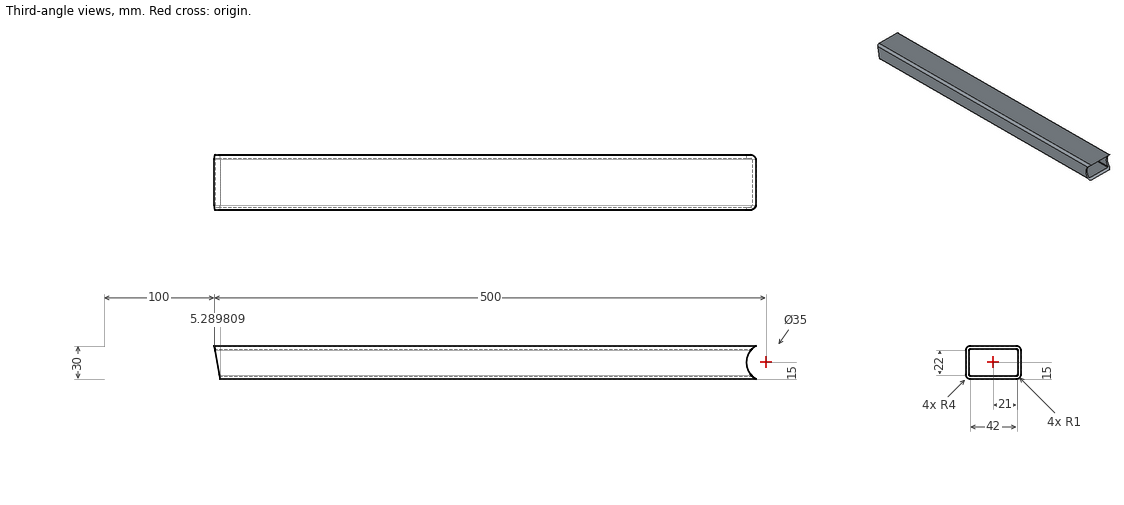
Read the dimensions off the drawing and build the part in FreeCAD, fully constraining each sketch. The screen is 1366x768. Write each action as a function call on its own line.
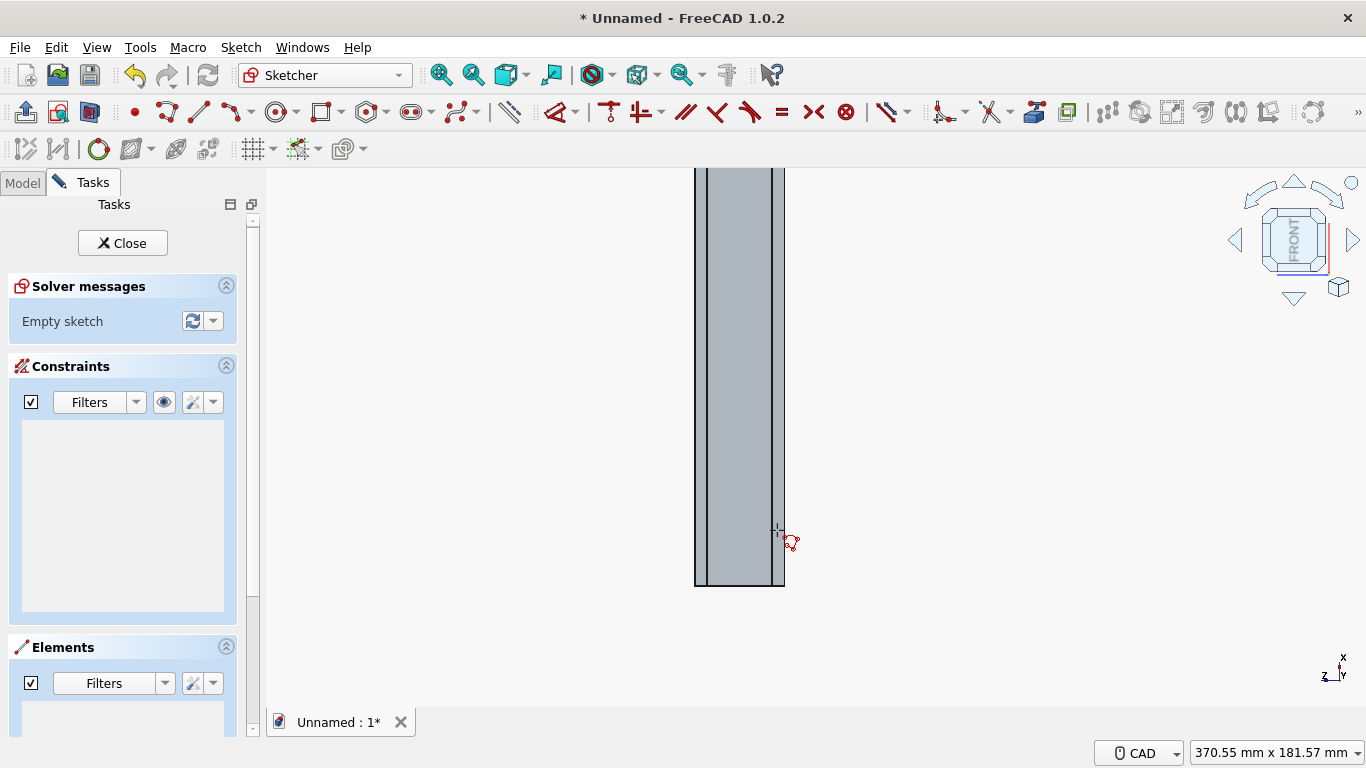
click(784, 274)
click(695, 289)
click(695, 586)
click(784, 586)
click(784, 275)
key(Escape)
key(Escape)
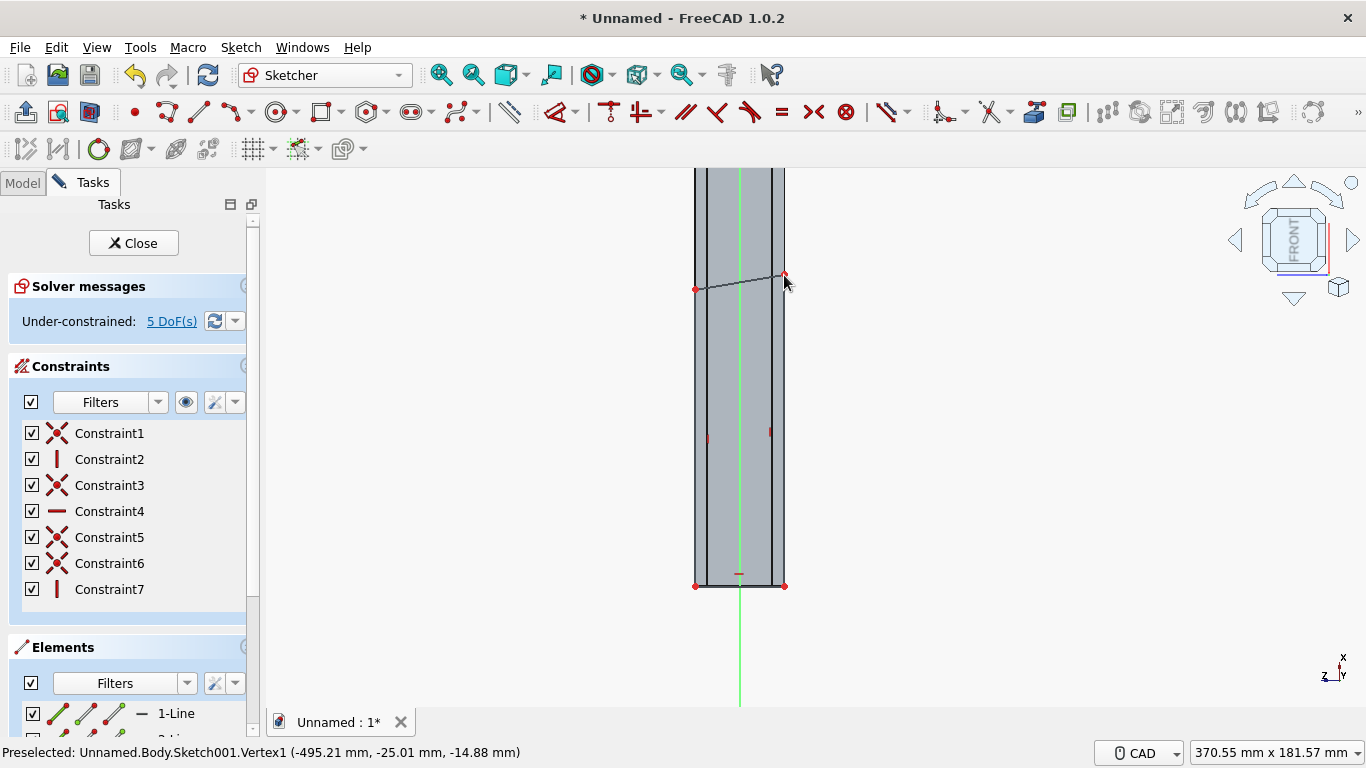
key(d)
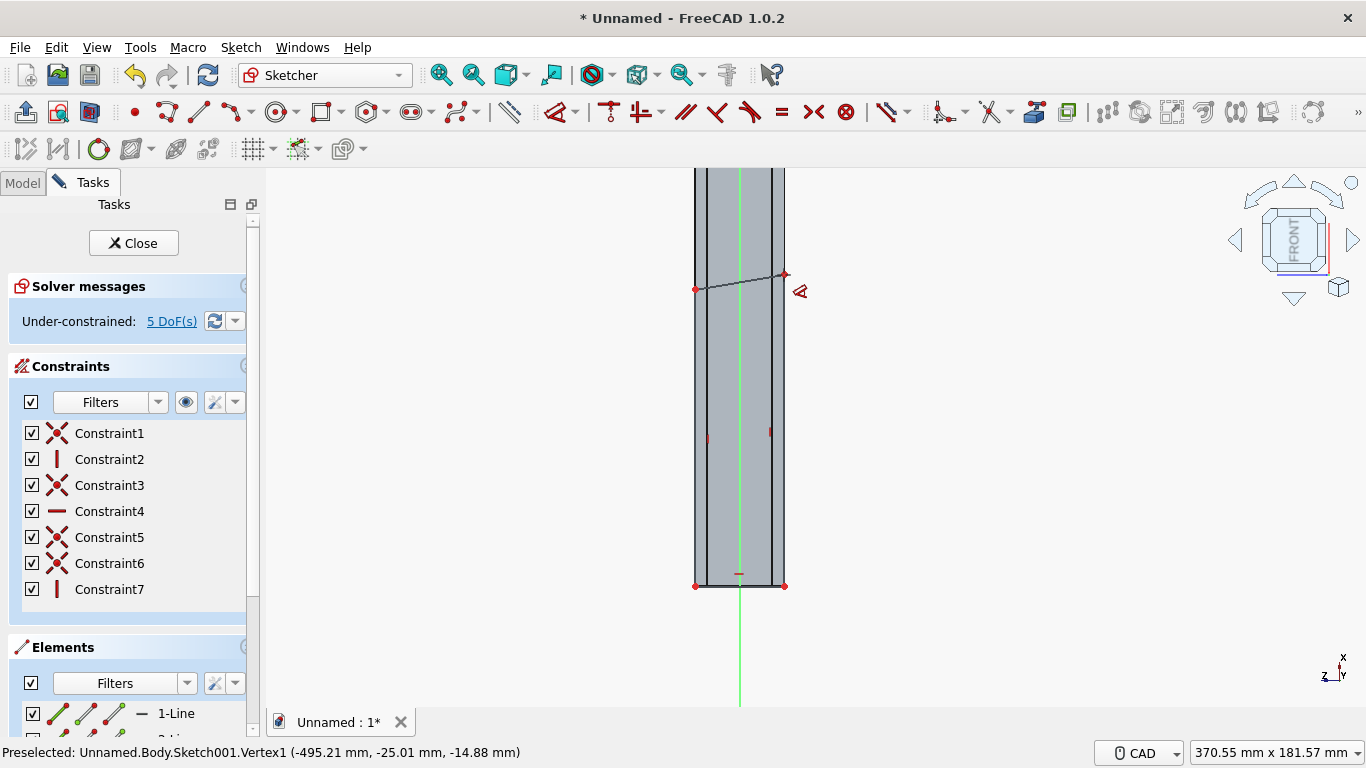
click(722, 587)
click(719, 621)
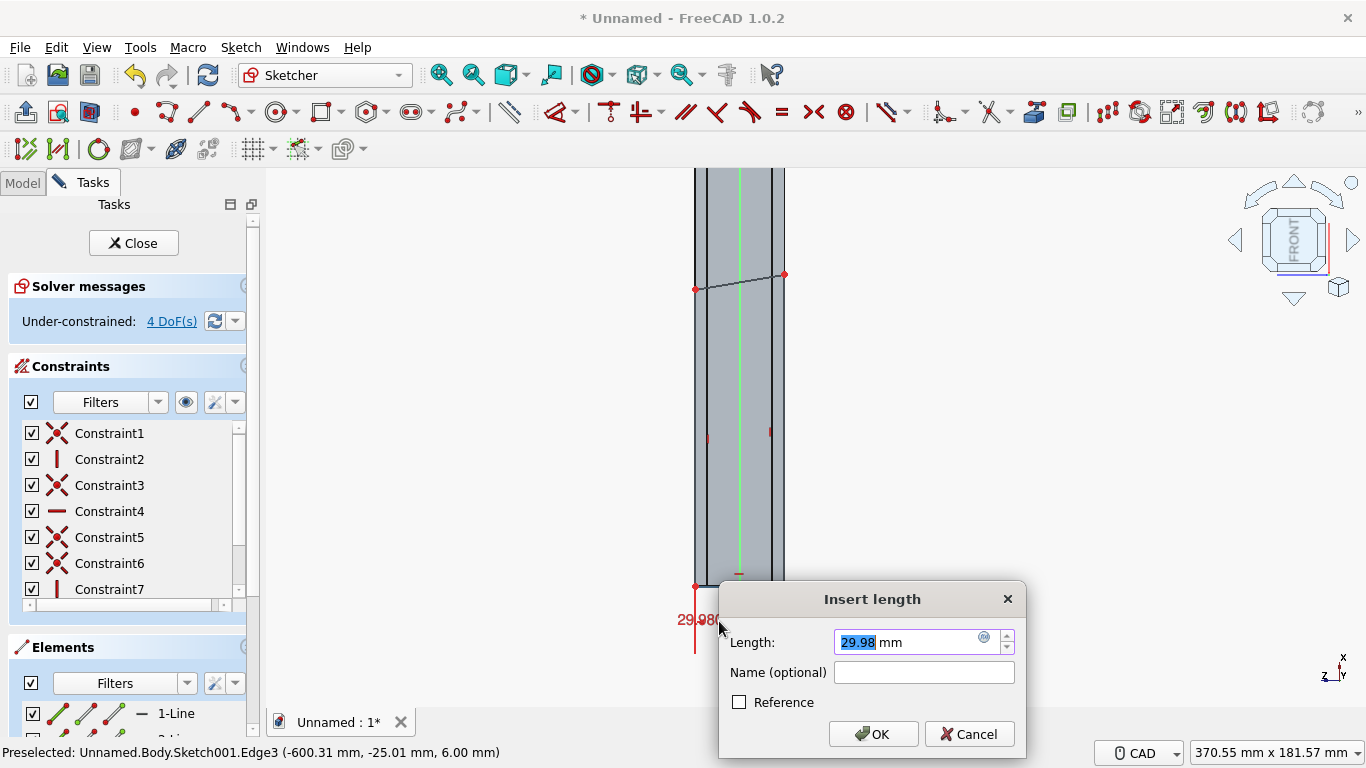
text(30)
key(Return)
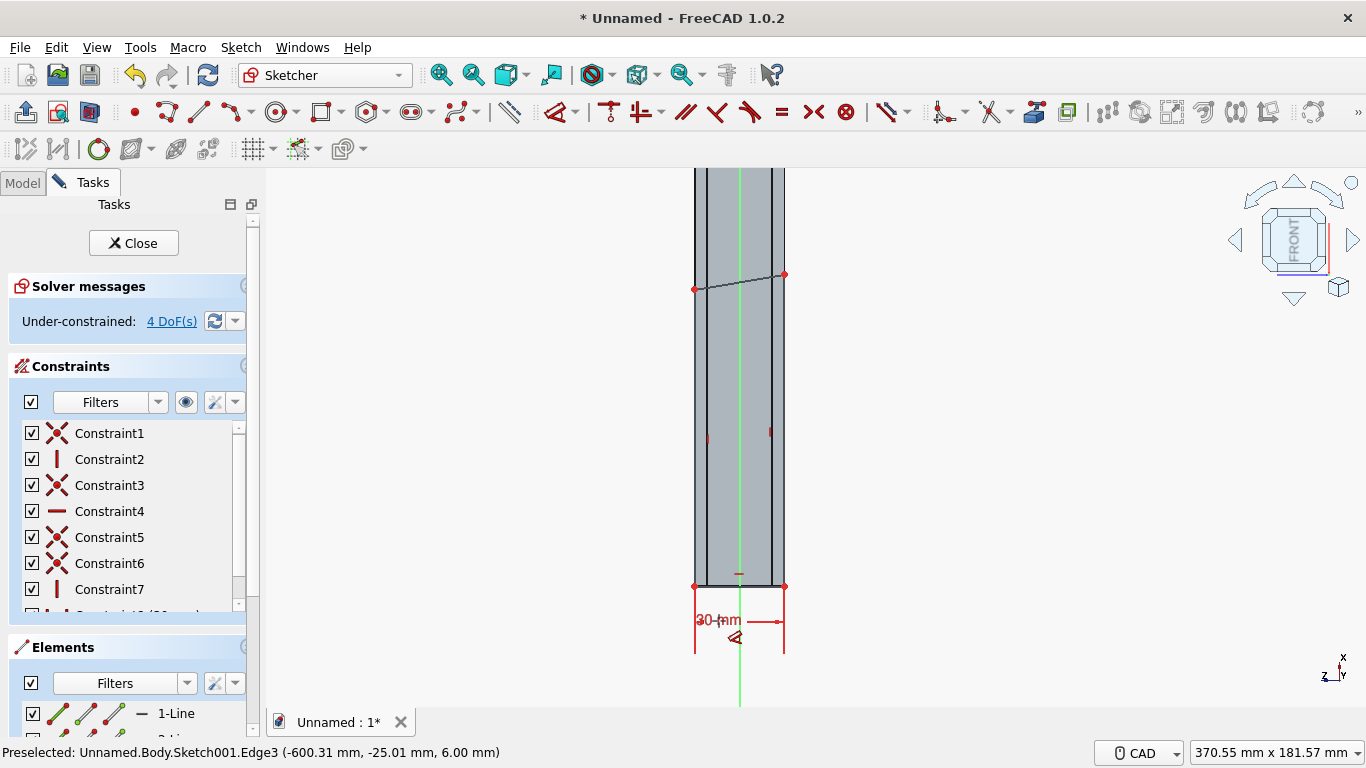
click(695, 379)
click(661, 438)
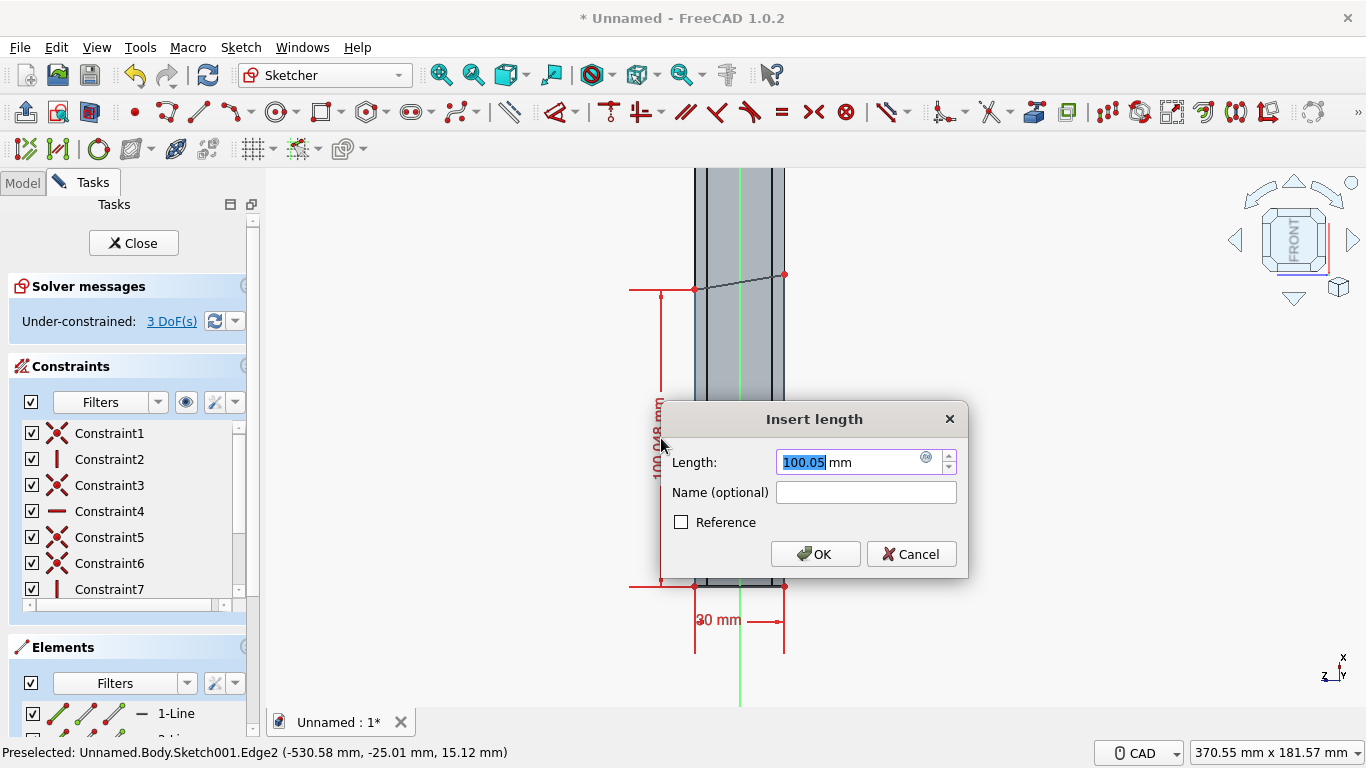
text(100)
key(Return)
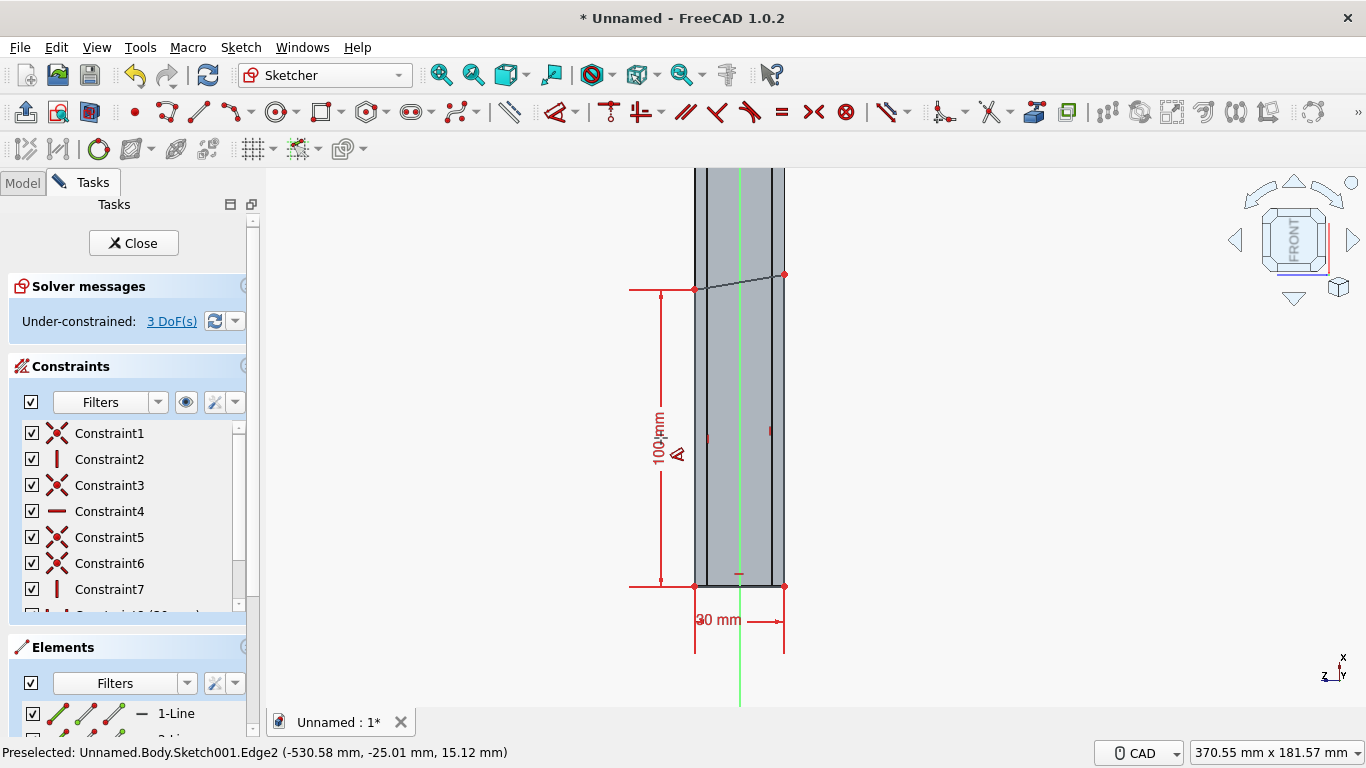
click(784, 275)
click(762, 309)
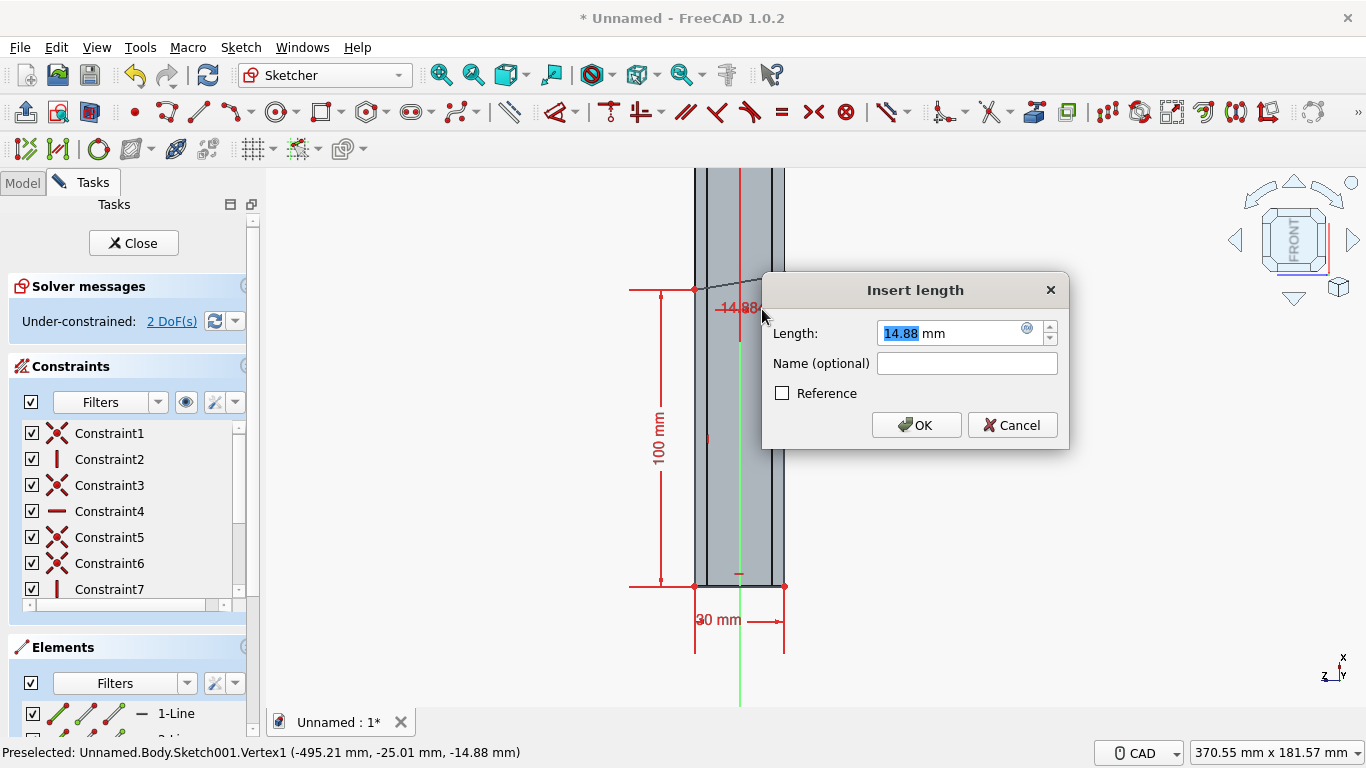
text(15)
key(Return)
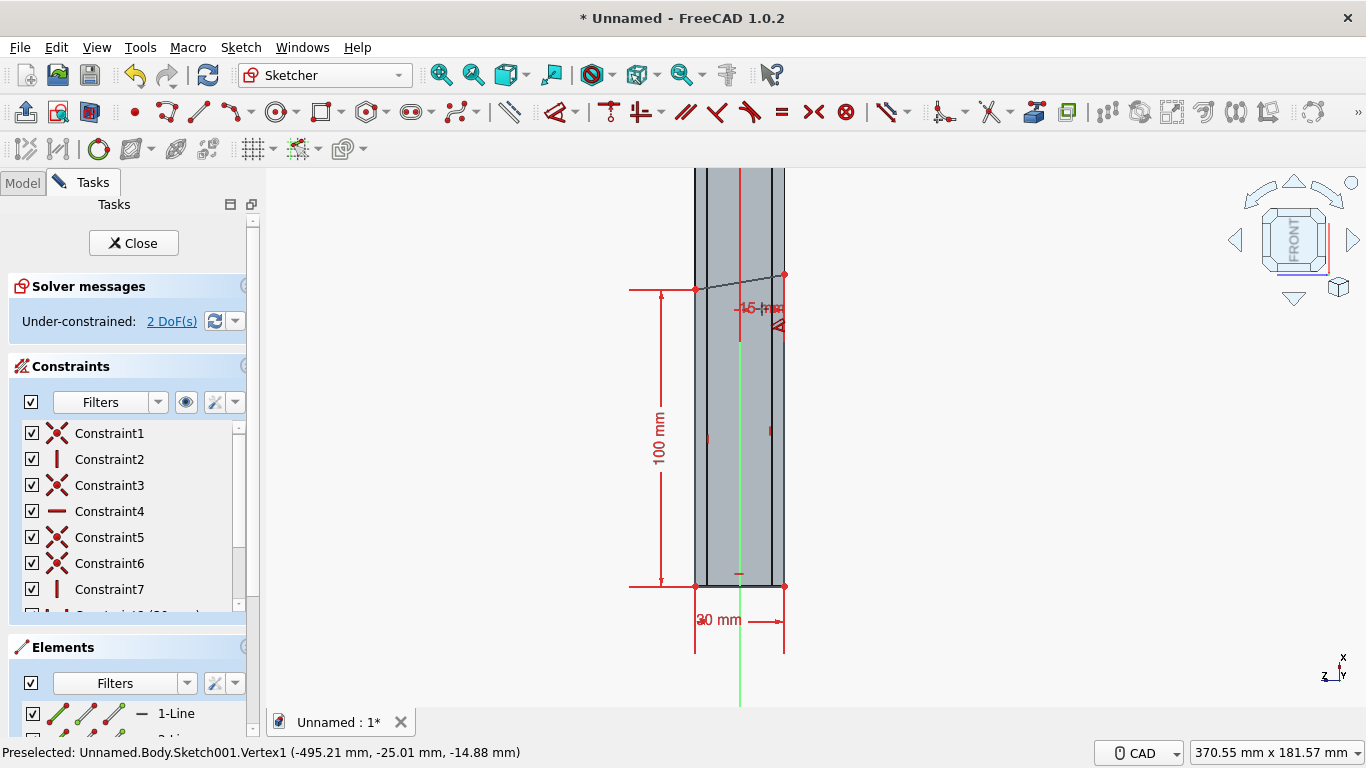
click(695, 290)
click(661, 243)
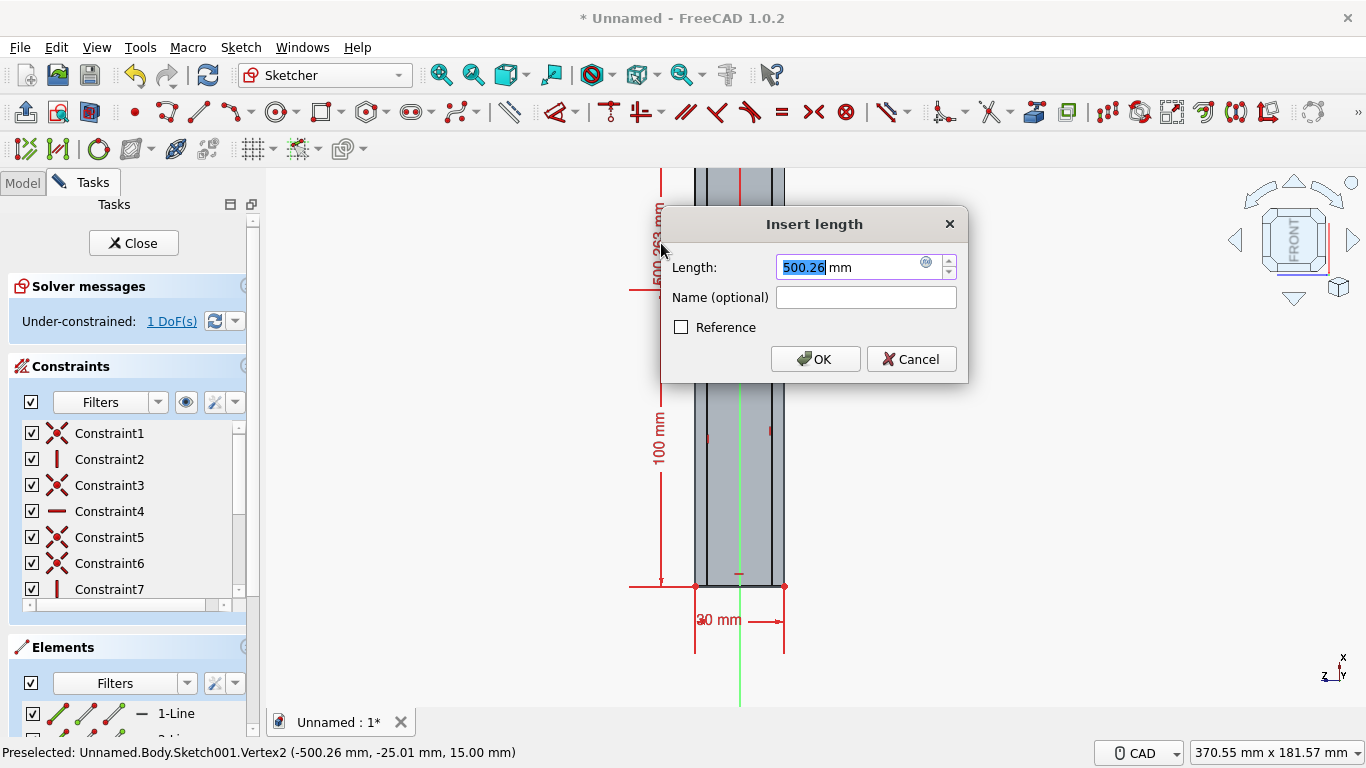
text(500)
key(Return)